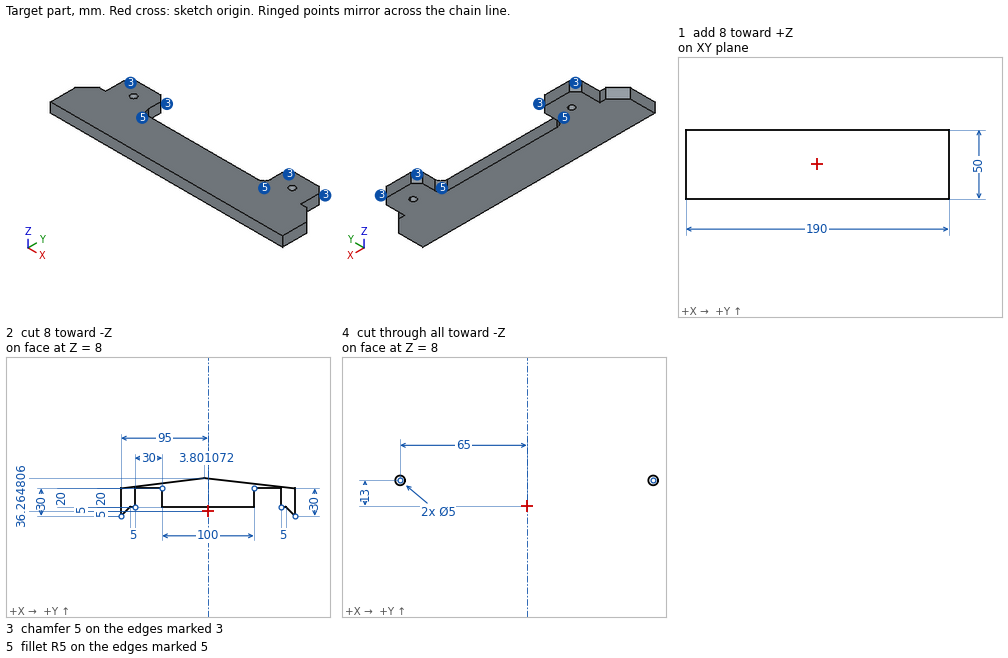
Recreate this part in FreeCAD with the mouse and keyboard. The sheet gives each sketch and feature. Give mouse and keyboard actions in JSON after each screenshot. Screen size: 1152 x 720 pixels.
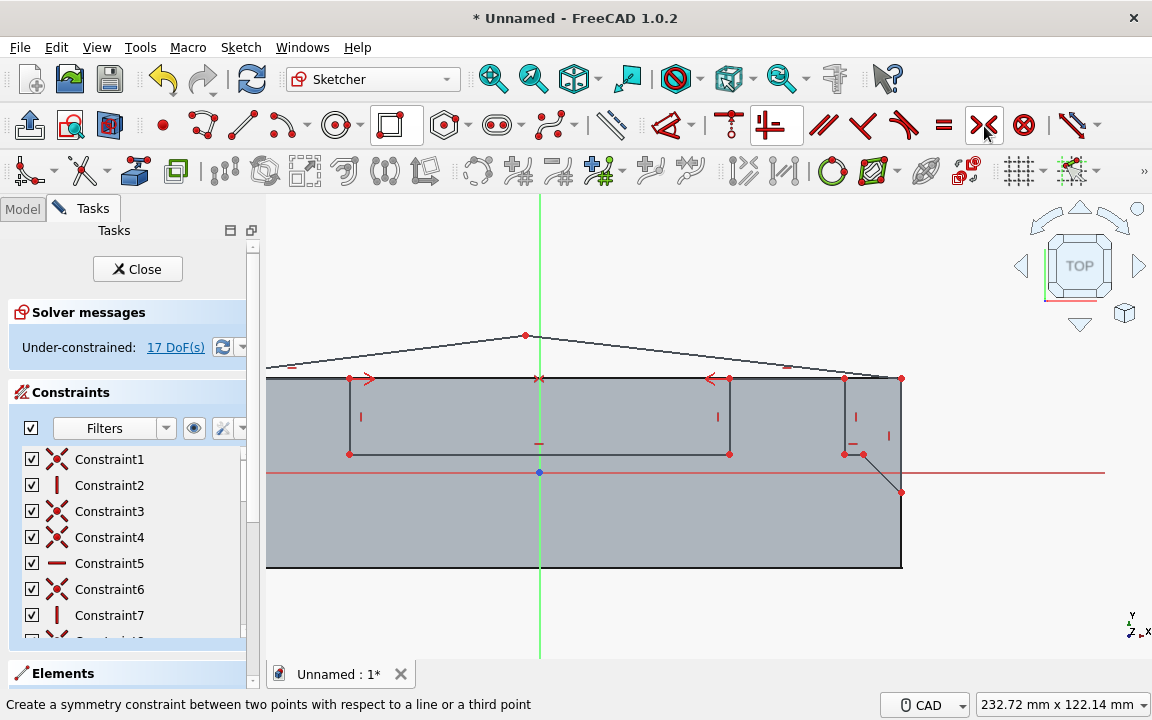
{"action": "scroll", "coordinate": [845, 454], "scroll_direction": "down", "scroll_amount": 2}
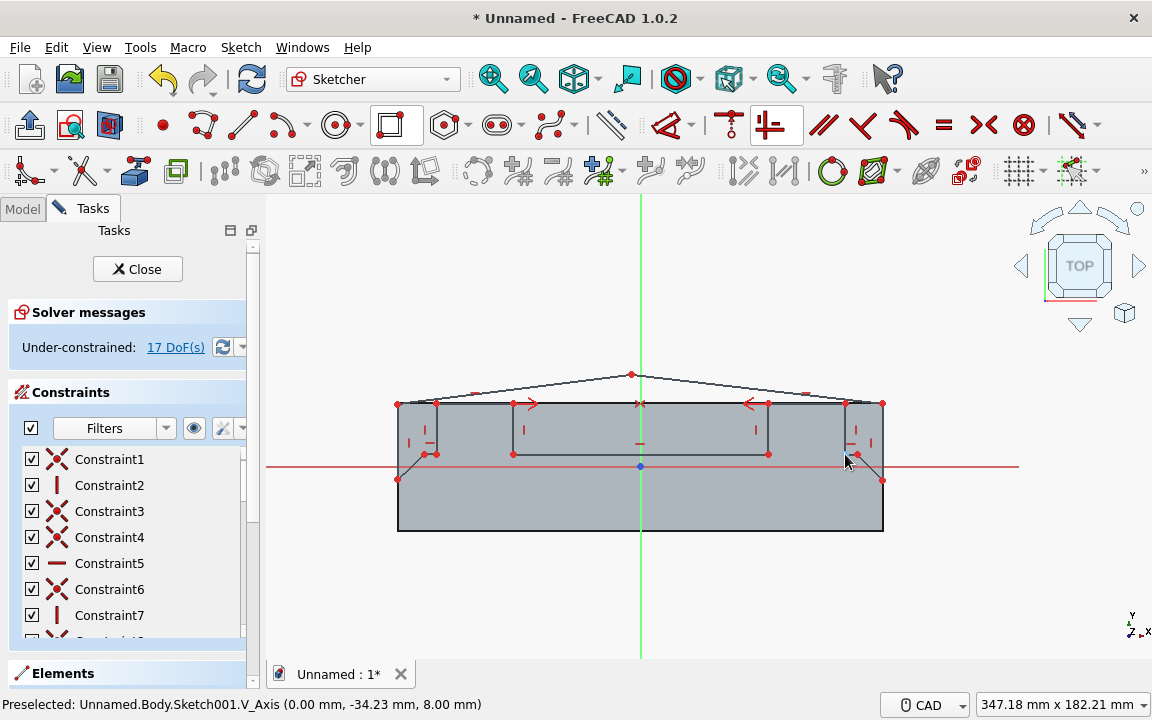
{"action": "left_click", "coordinate": [437, 454]}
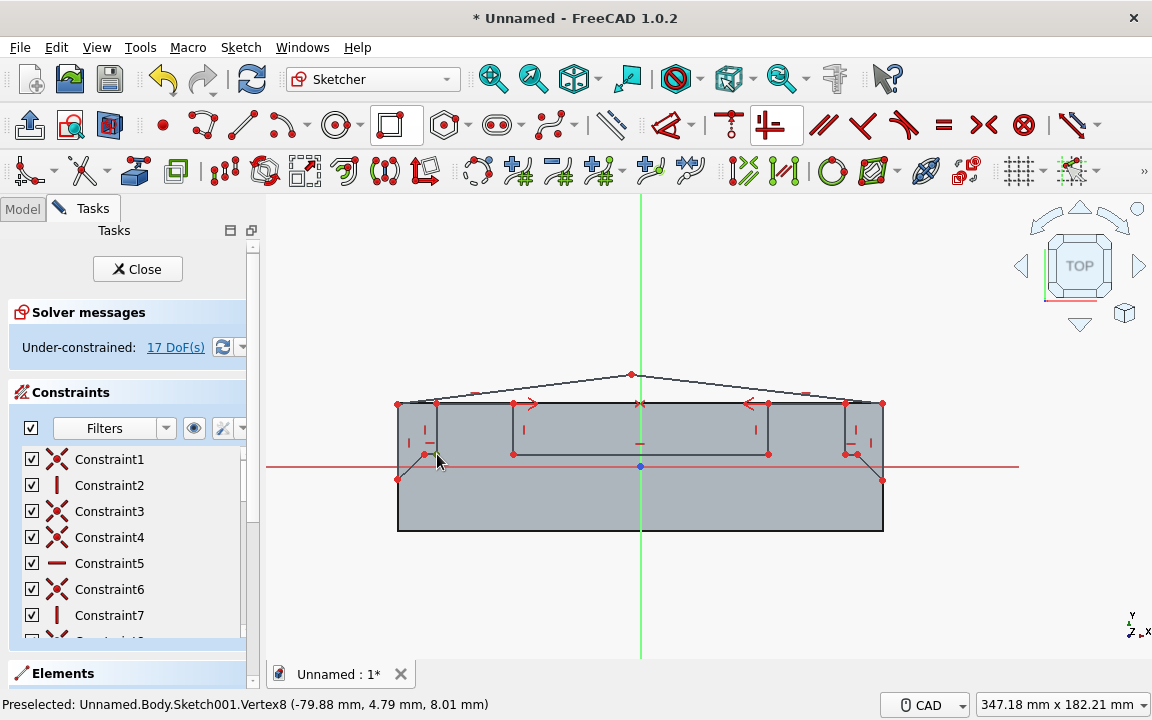
{"action": "left_click", "coordinate": [845, 455]}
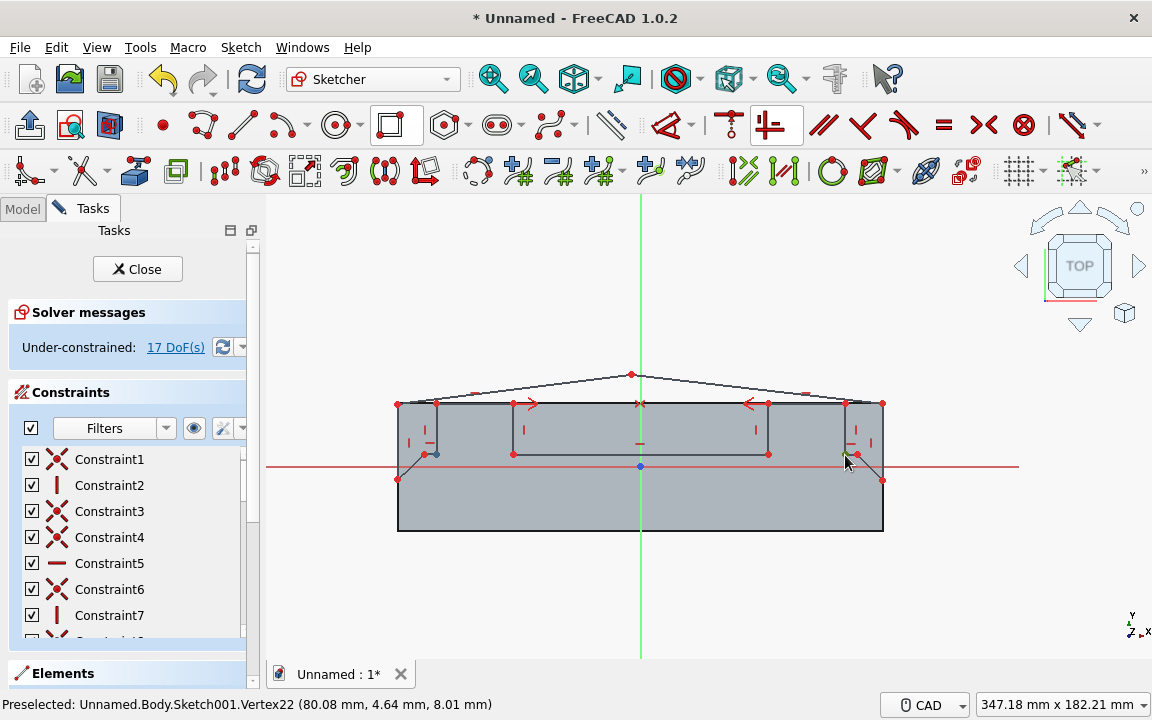
{"action": "left_click", "coordinate": [641, 602]}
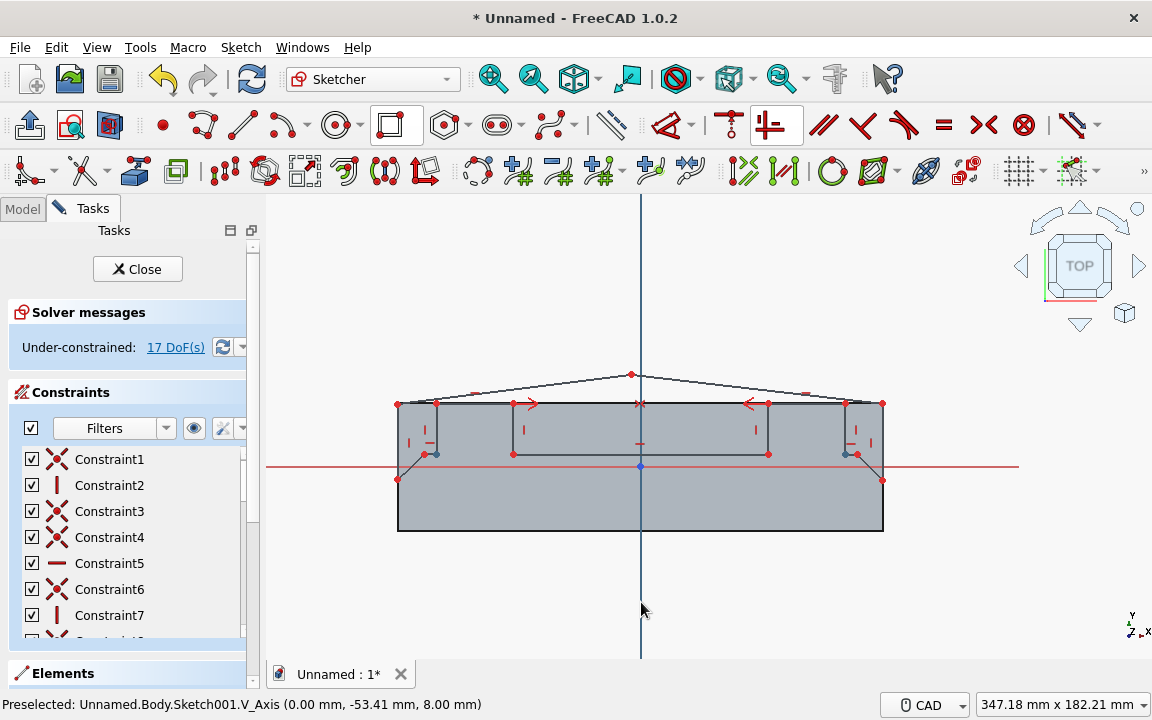
{"action": "left_click", "coordinate": [984, 126]}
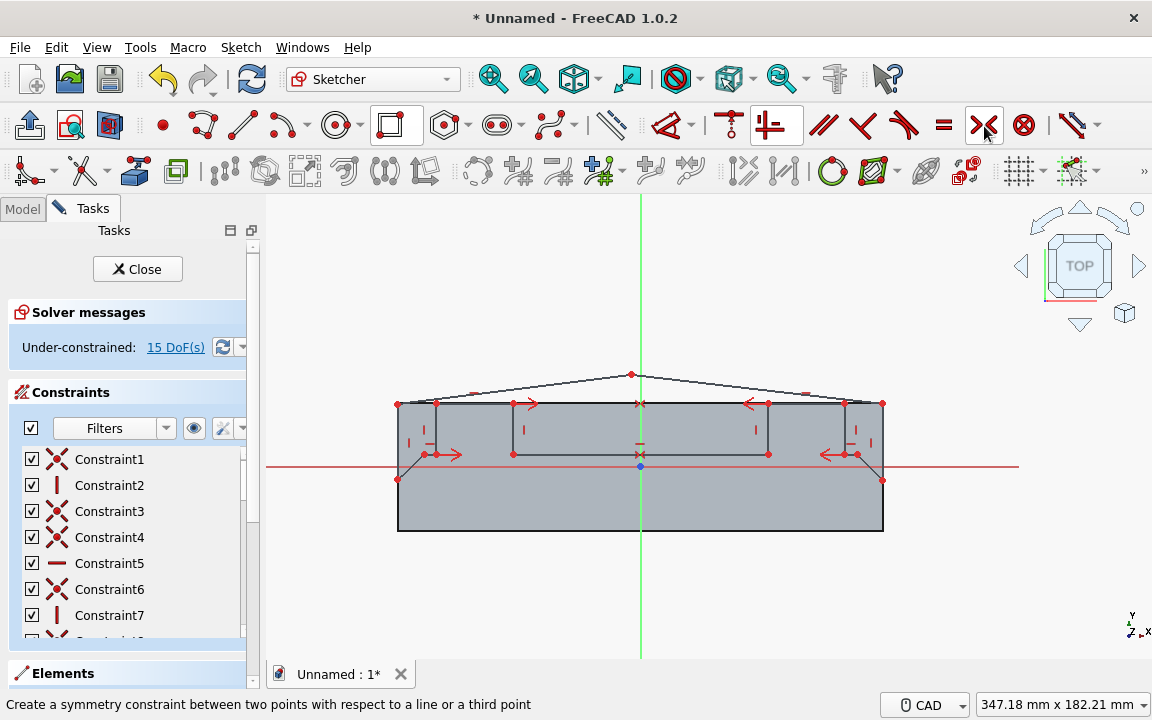
{"action": "left_click", "coordinate": [398, 480]}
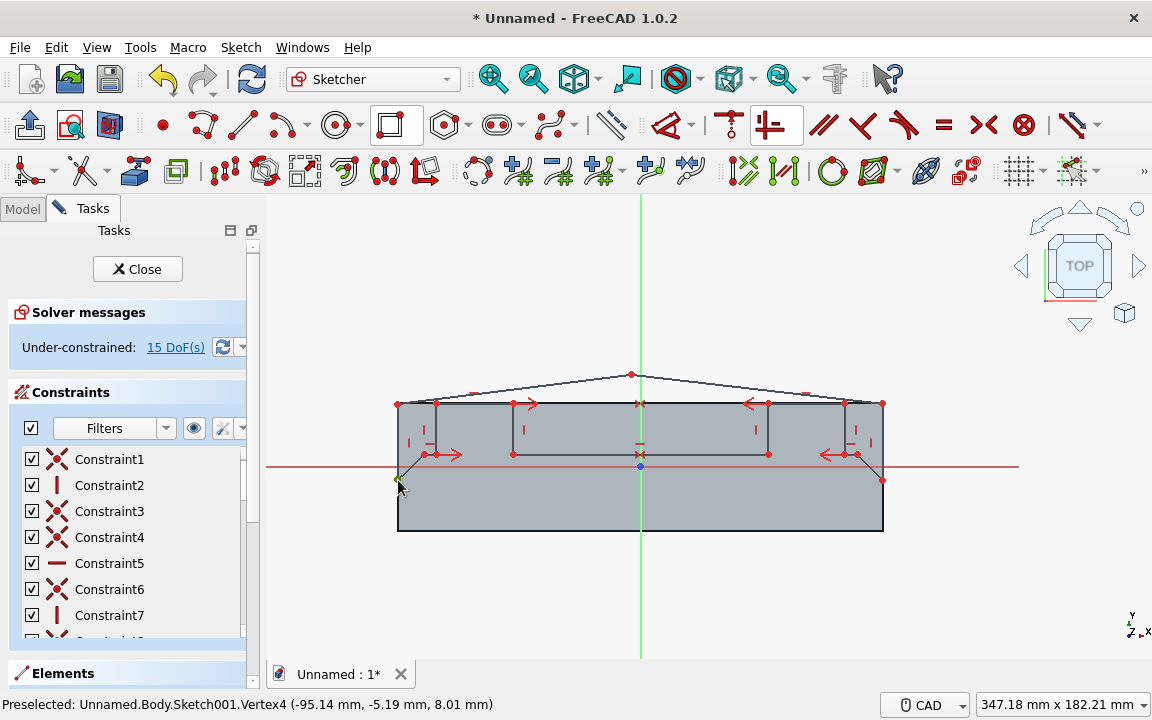
{"action": "left_click", "coordinate": [883, 480]}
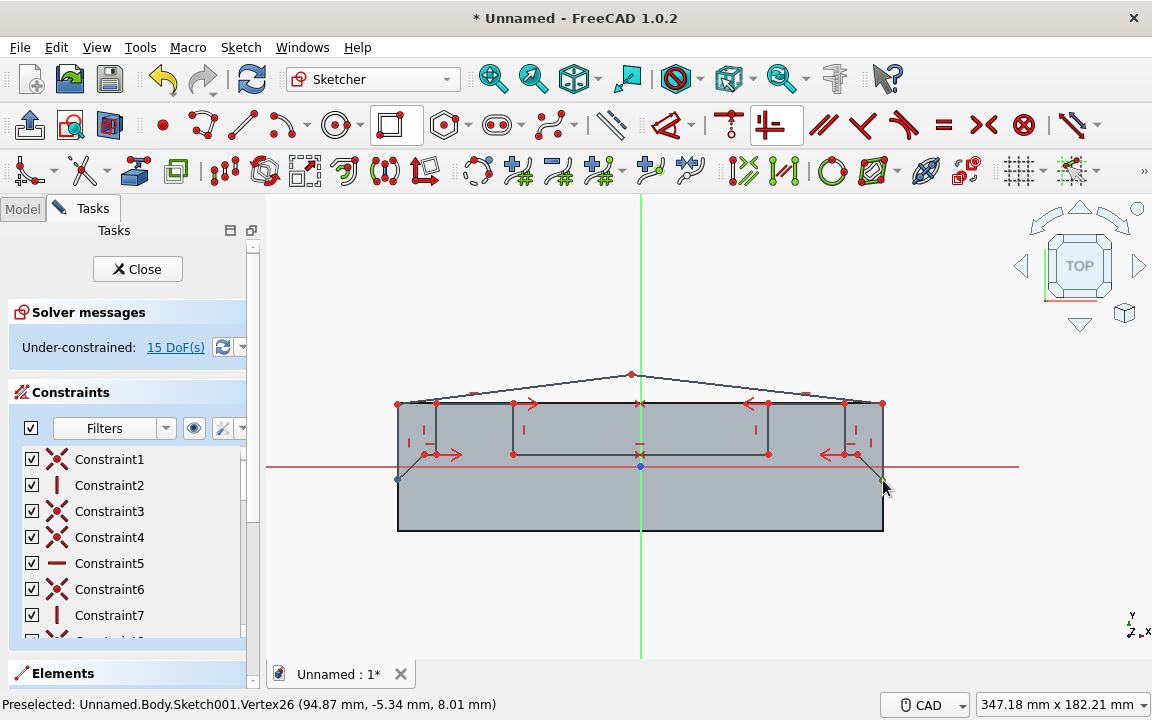
{"action": "left_click", "coordinate": [641, 602]}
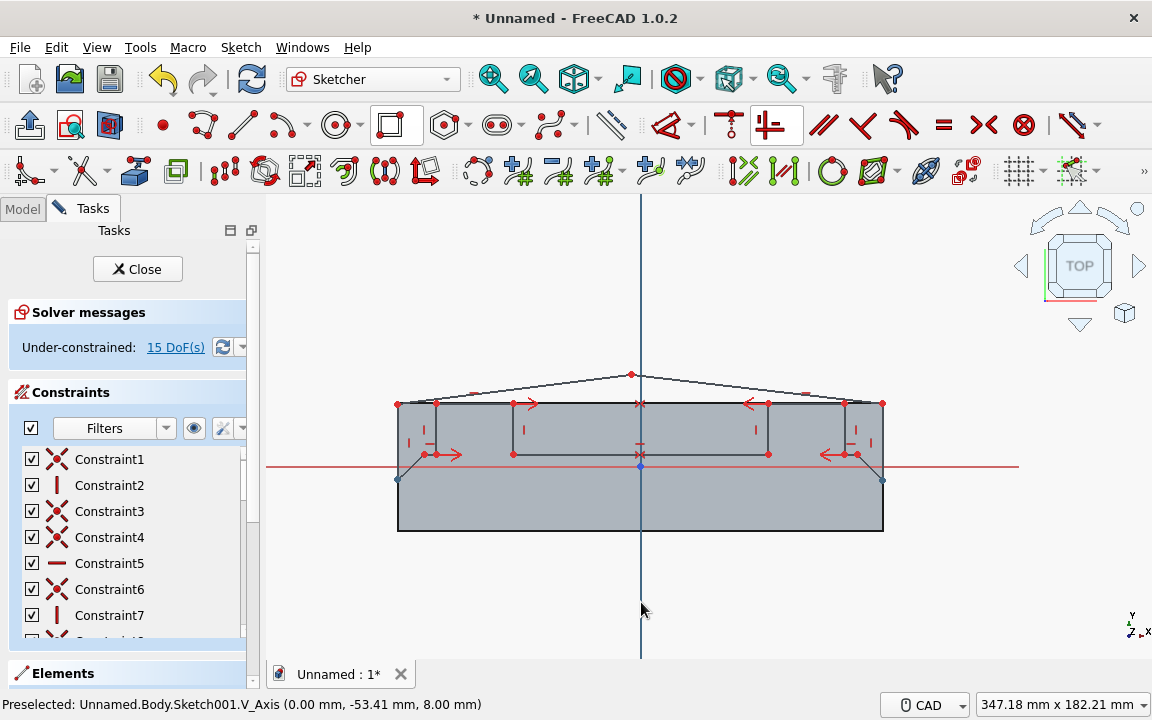
{"action": "left_click", "coordinate": [984, 126]}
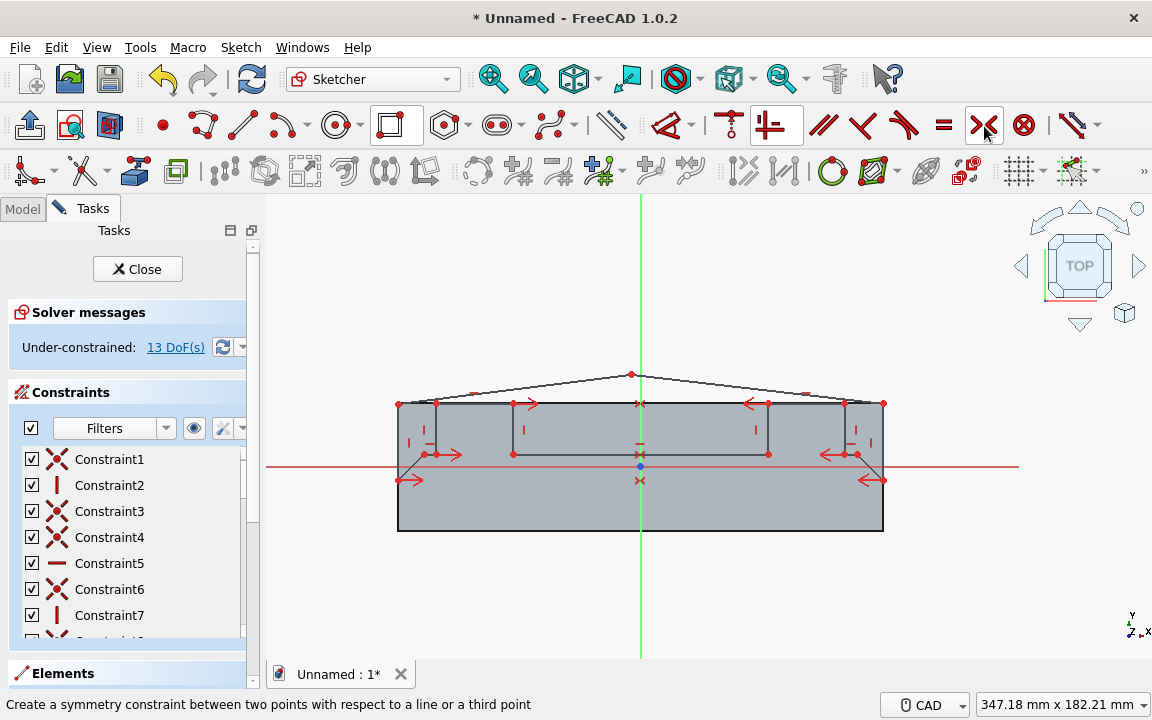
{"action": "left_click", "coordinate": [666, 126]}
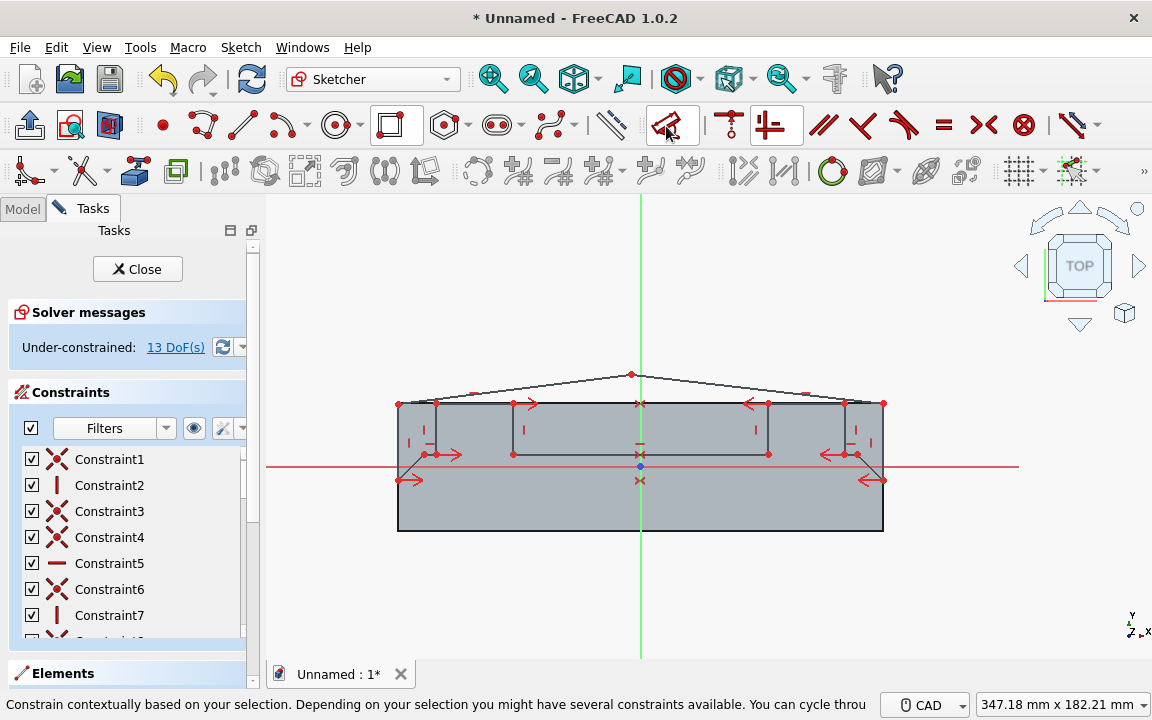
{"action": "scroll", "coordinate": [430, 455], "scroll_direction": "up", "scroll_amount": 6}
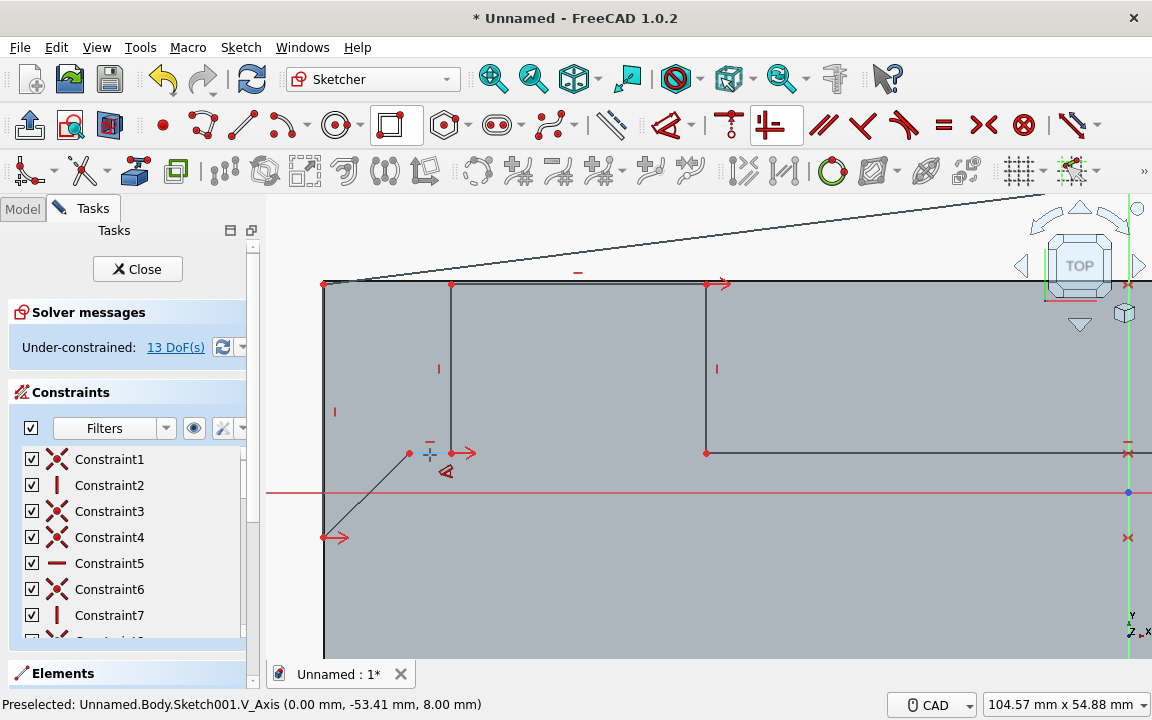
{"action": "left_click", "coordinate": [430, 453]}
{"action": "left_click", "coordinate": [430, 419]}